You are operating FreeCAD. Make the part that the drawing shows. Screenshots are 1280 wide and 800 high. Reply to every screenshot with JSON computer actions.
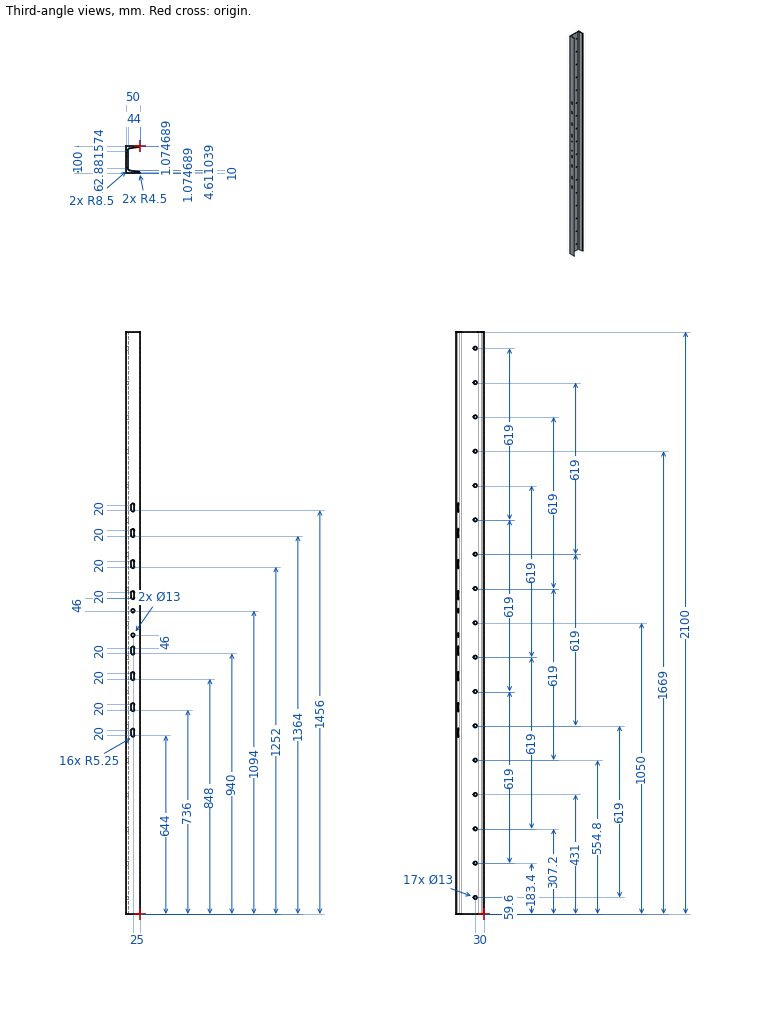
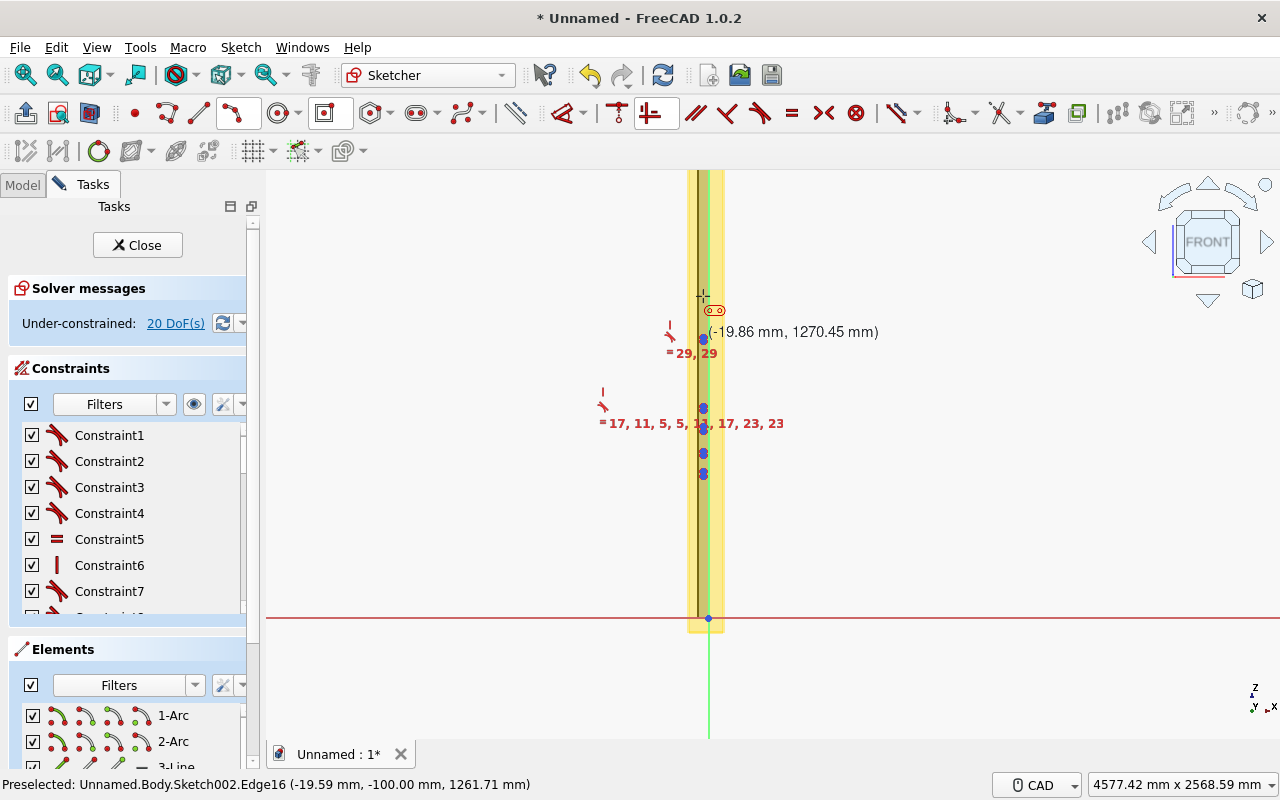
{"action": "scroll", "coordinate": [703, 296], "scroll_direction": "up", "scroll_amount": 6}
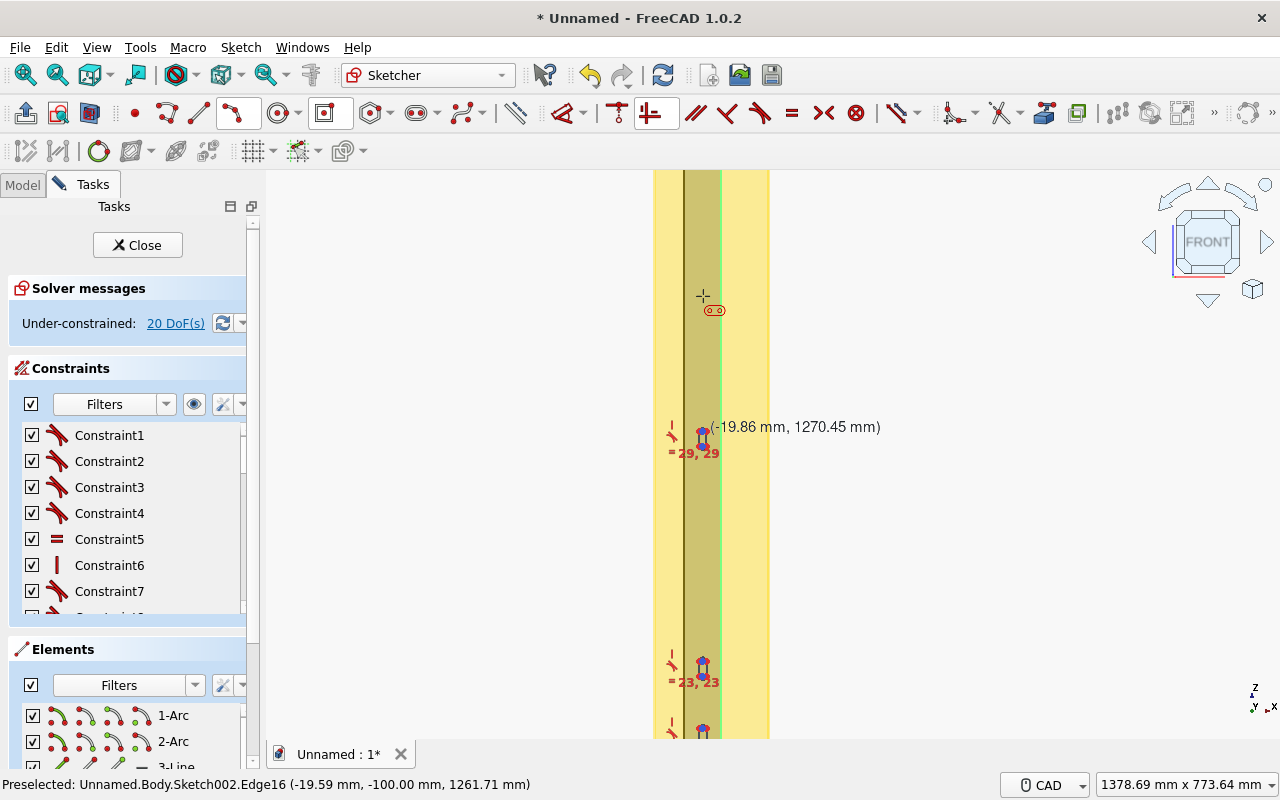
{"action": "left_click", "coordinate": [703, 295]}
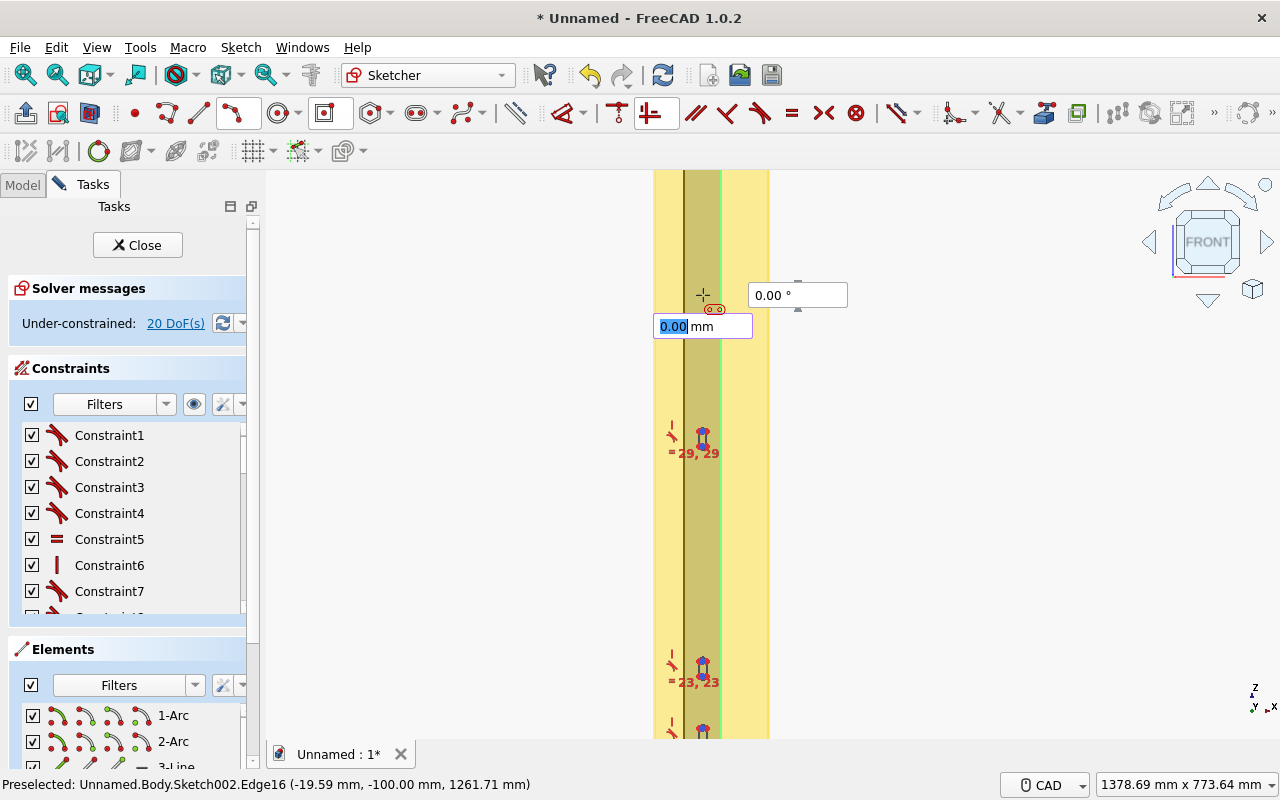
{"action": "left_click", "coordinate": [703, 281]}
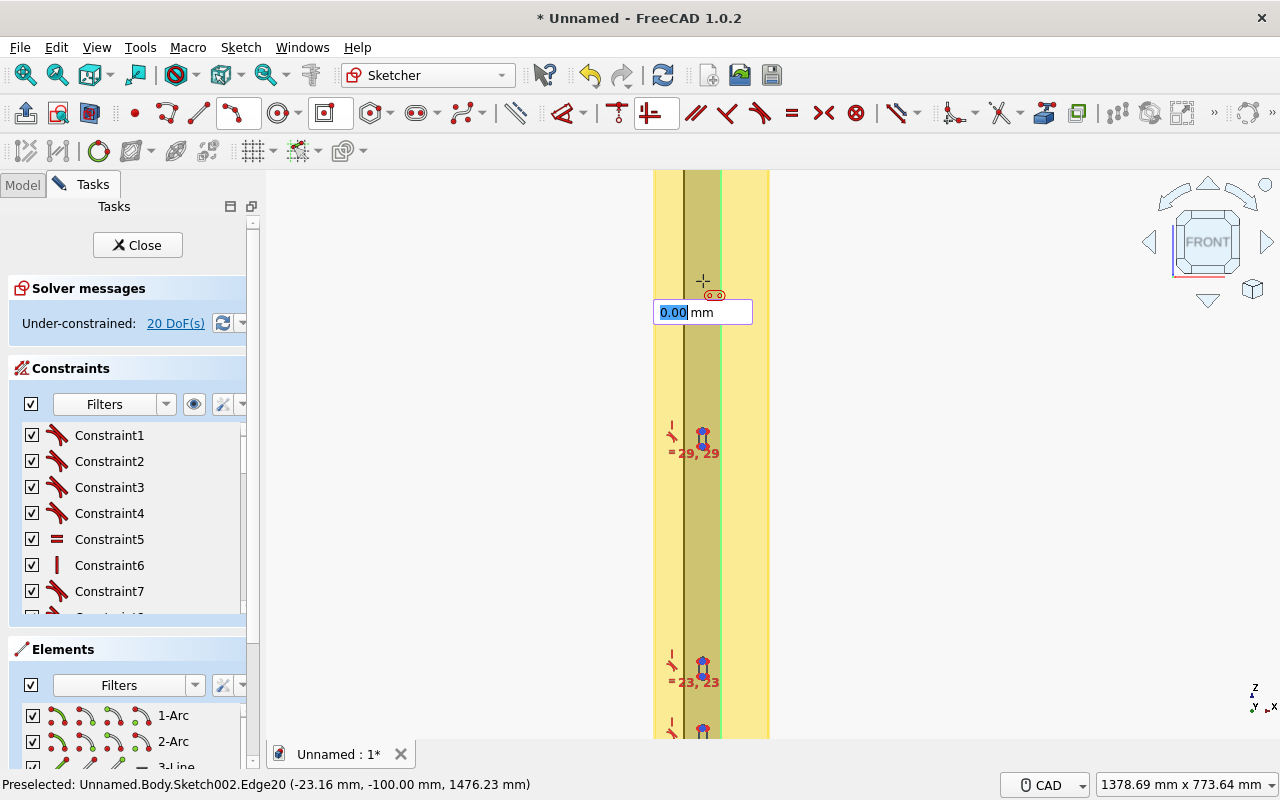
{"action": "scroll", "coordinate": [707, 288], "scroll_direction": "up", "scroll_amount": 8}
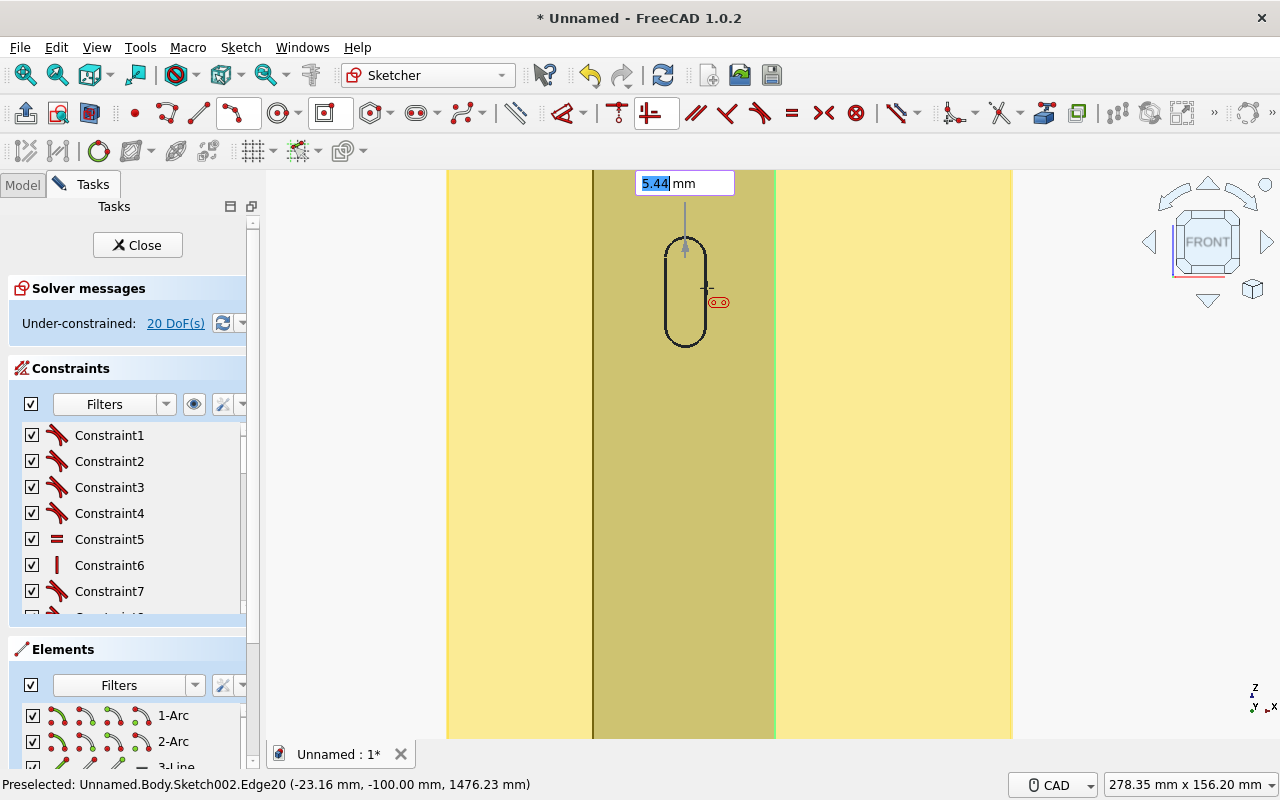
{"action": "left_click", "coordinate": [703, 287]}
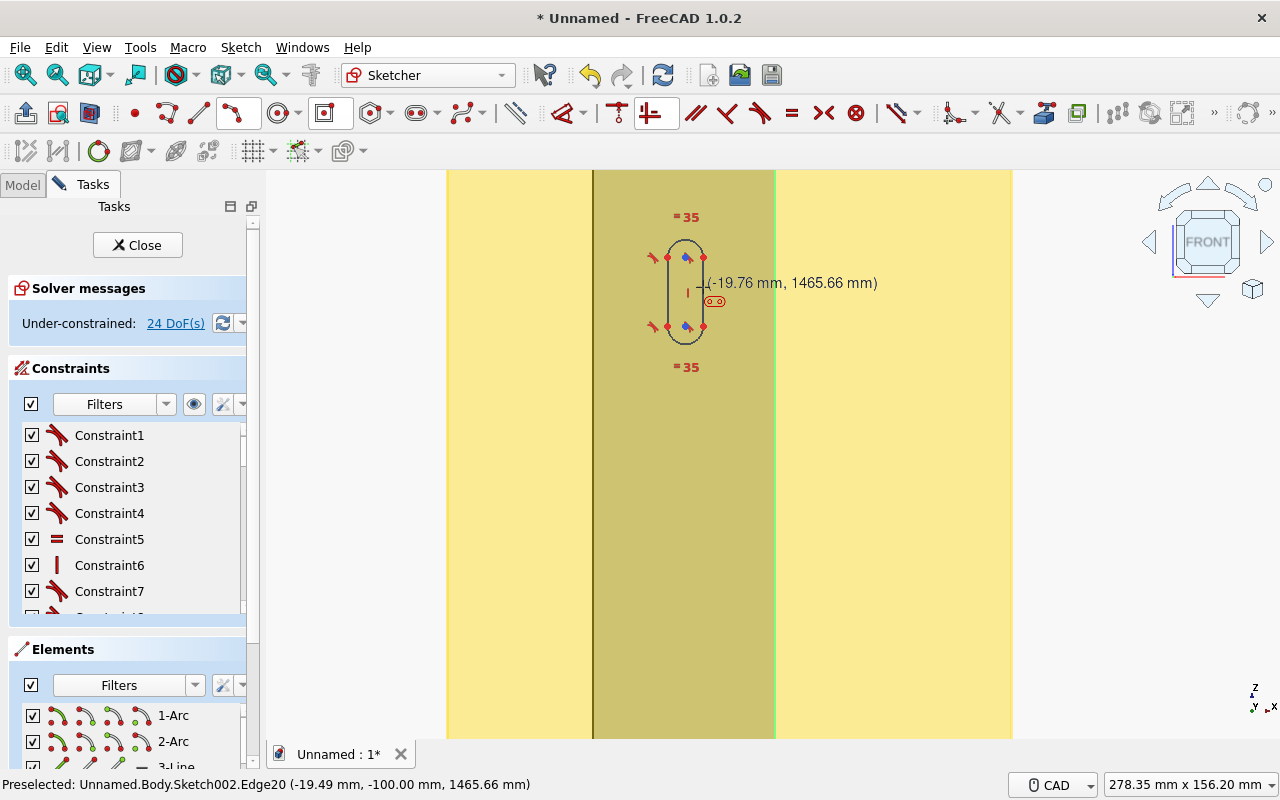
{"action": "scroll", "coordinate": [704, 294], "scroll_direction": "down", "scroll_amount": 14}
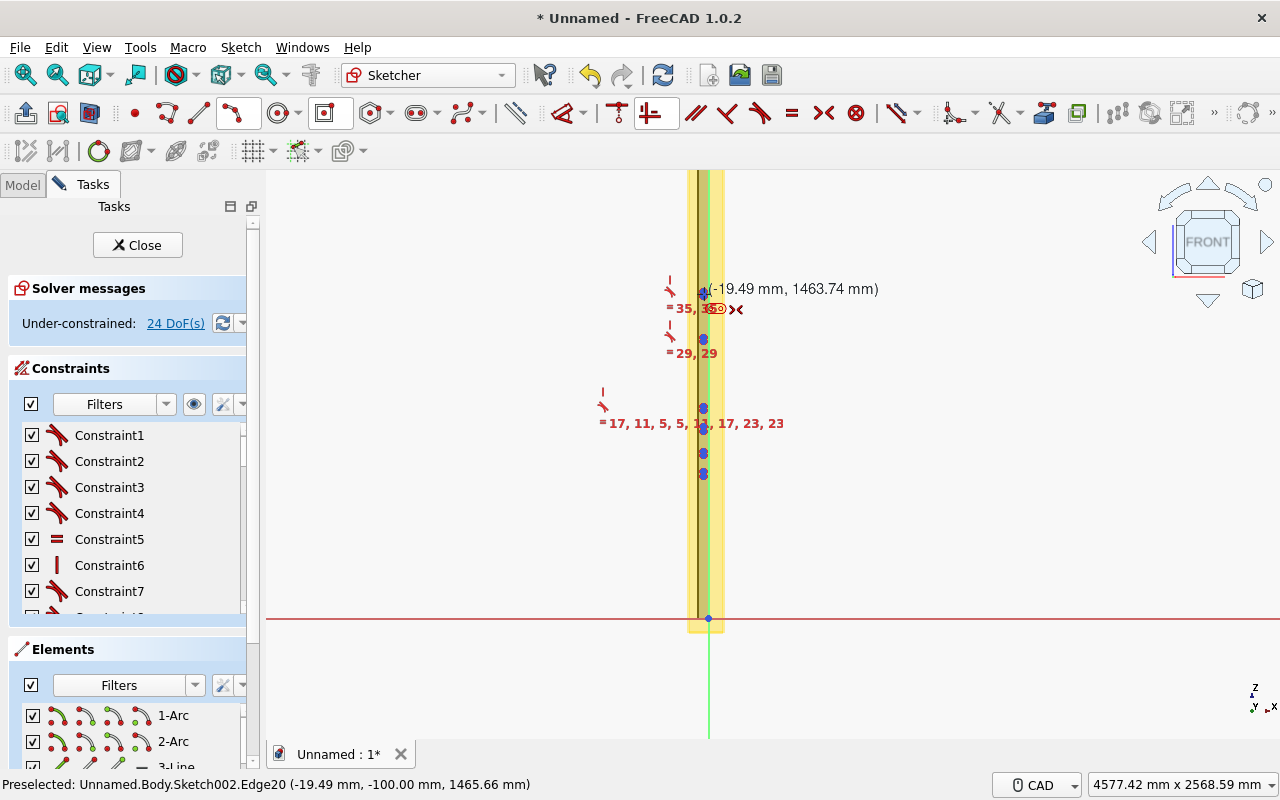
{"action": "scroll", "coordinate": [703, 316], "scroll_direction": "up", "scroll_amount": 6}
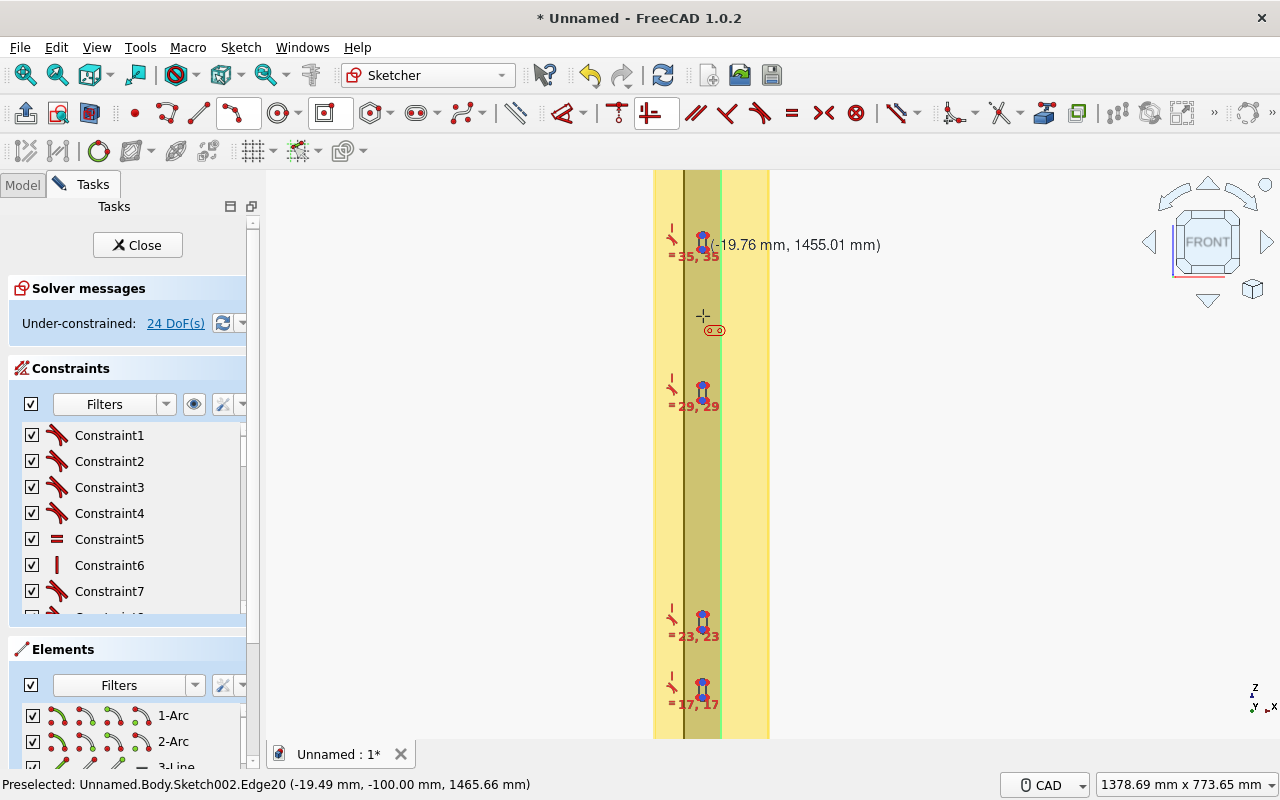
{"action": "left_click", "coordinate": [703, 317]}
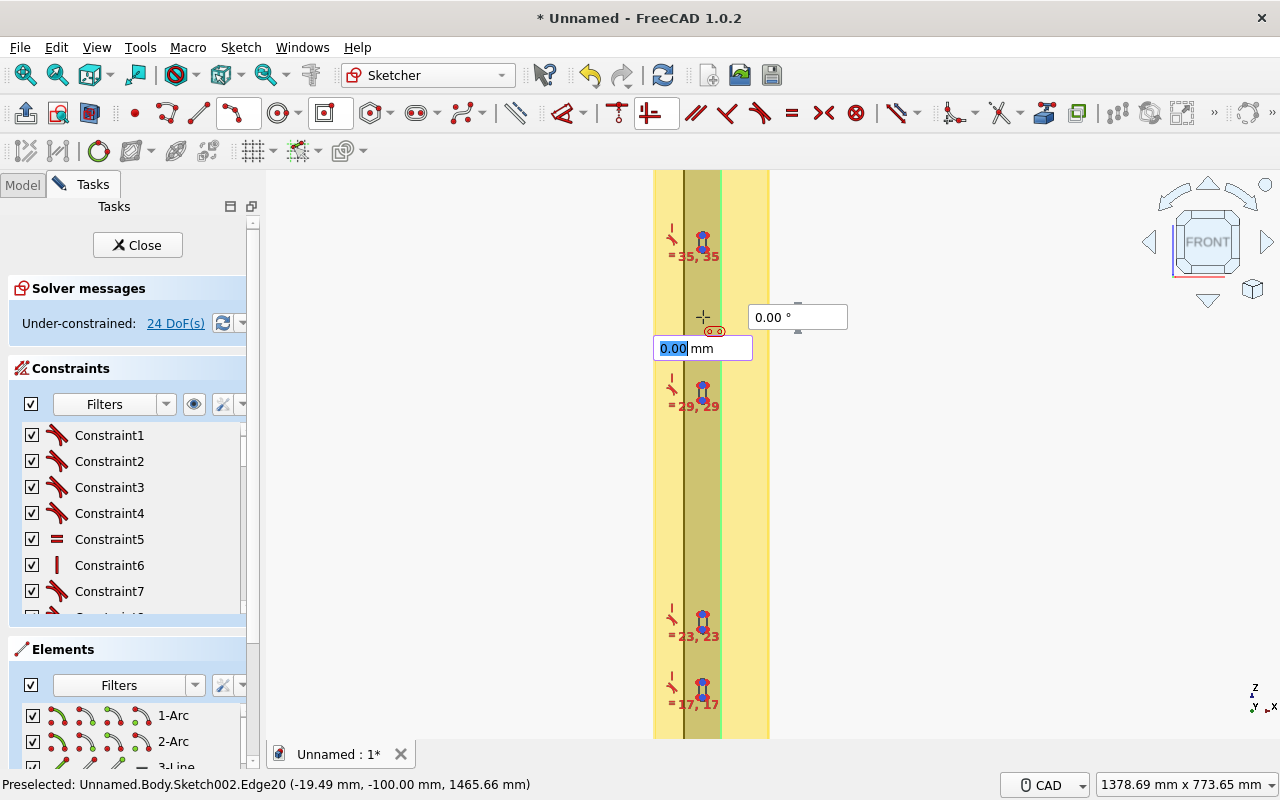
{"action": "left_click", "coordinate": [703, 302]}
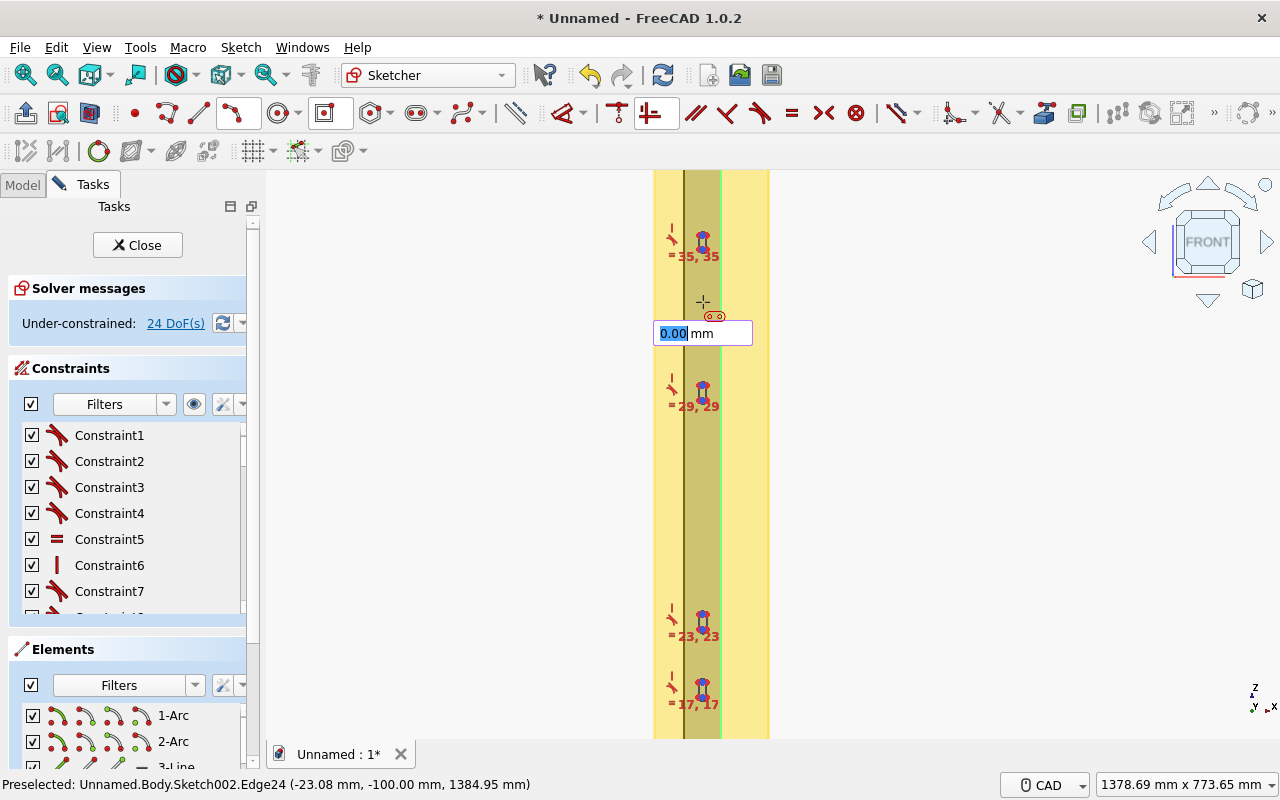
{"action": "scroll", "coordinate": [706, 309], "scroll_direction": "up", "scroll_amount": 8}